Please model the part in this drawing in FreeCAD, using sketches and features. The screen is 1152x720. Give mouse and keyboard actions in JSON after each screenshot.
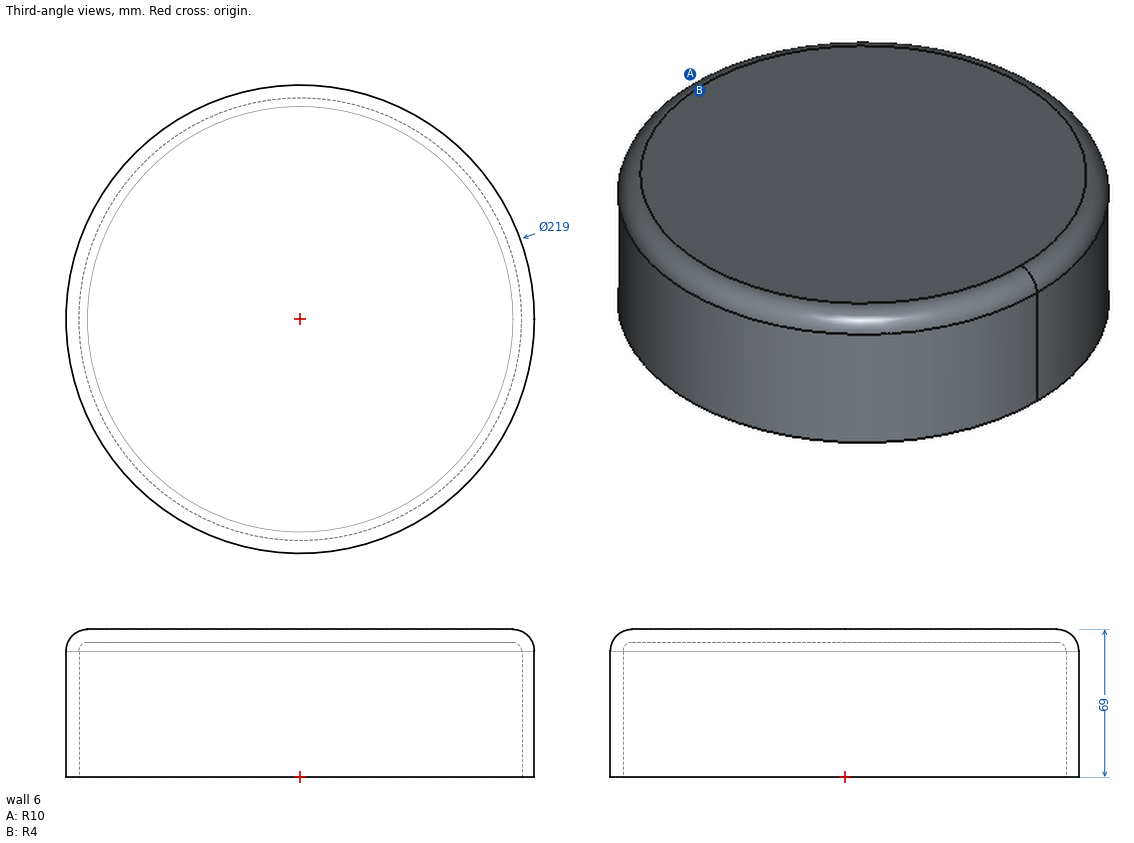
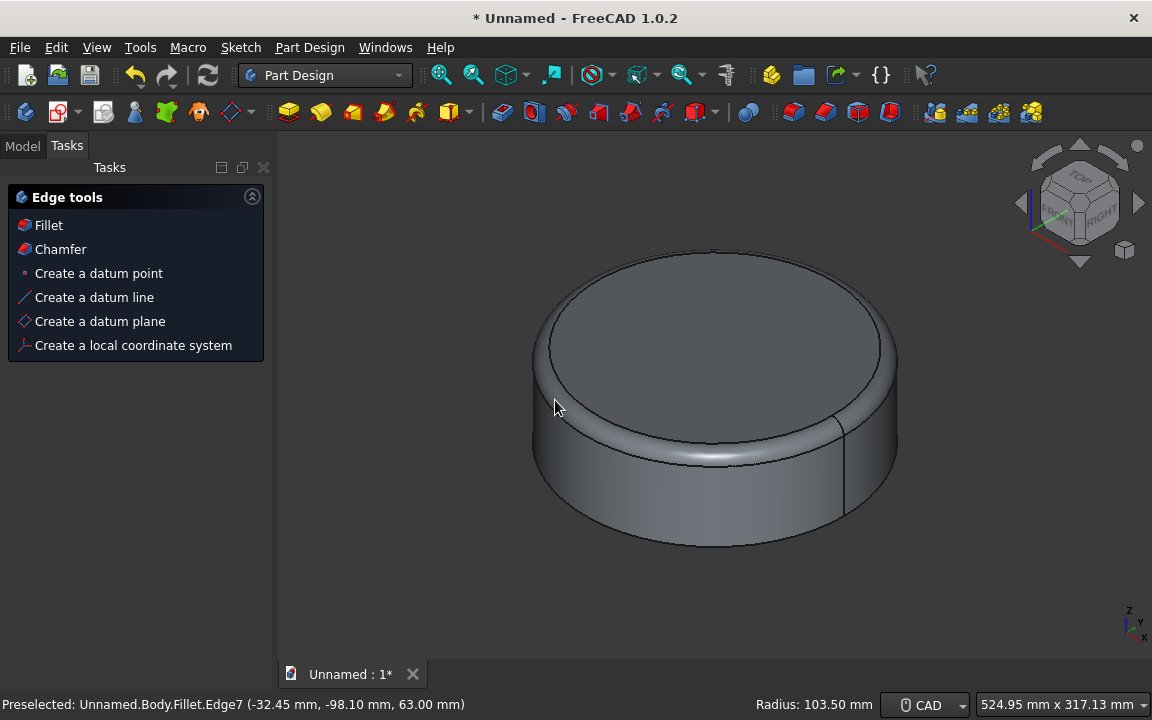
{"action": "left_click", "coordinate": [794, 112]}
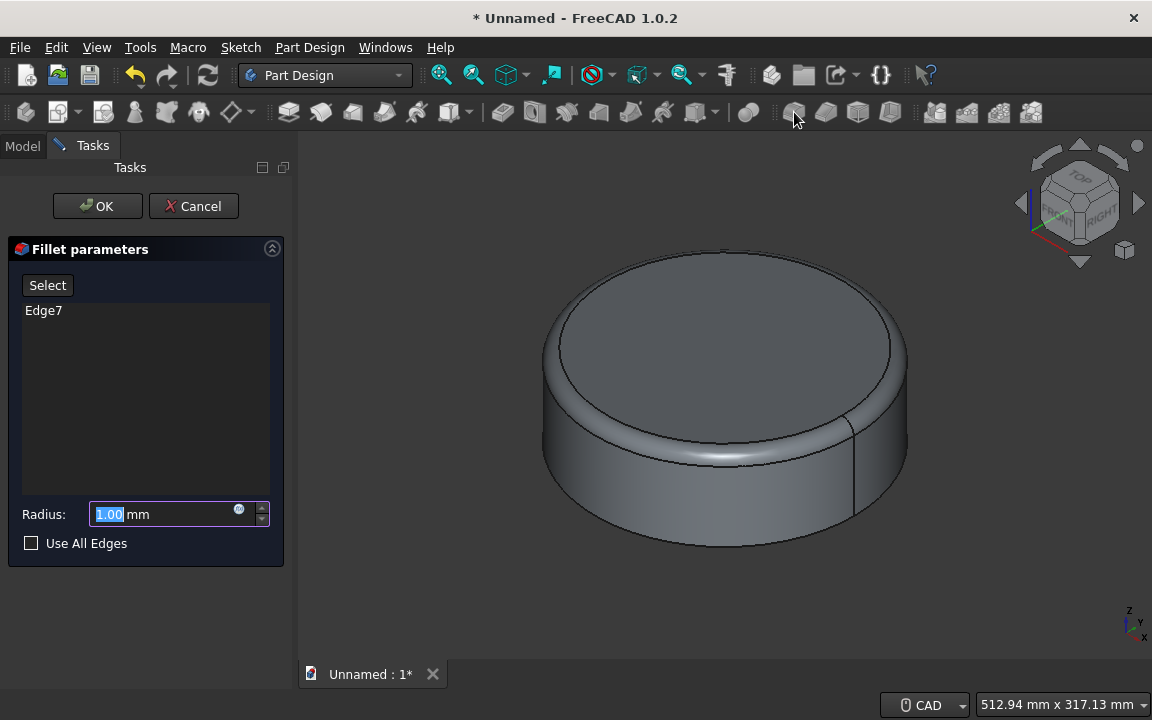
{"action": "type", "text": "4"}
{"action": "key", "text": "Tab"}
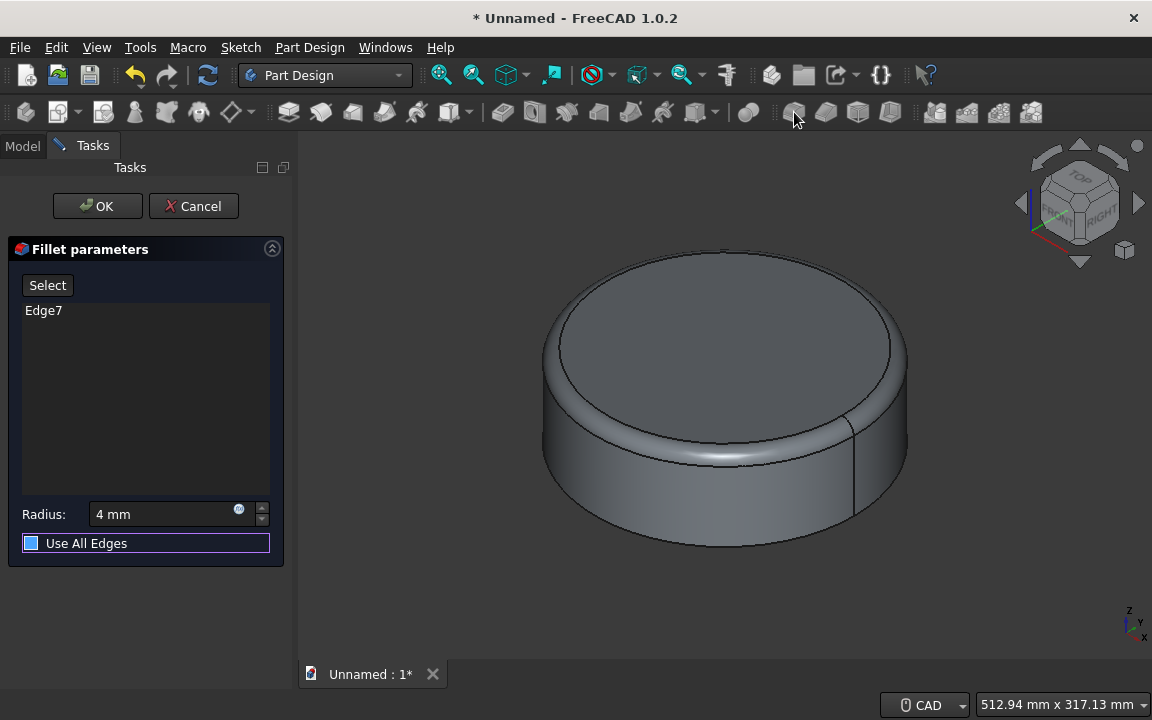
{"action": "left_click", "coordinate": [98, 206]}